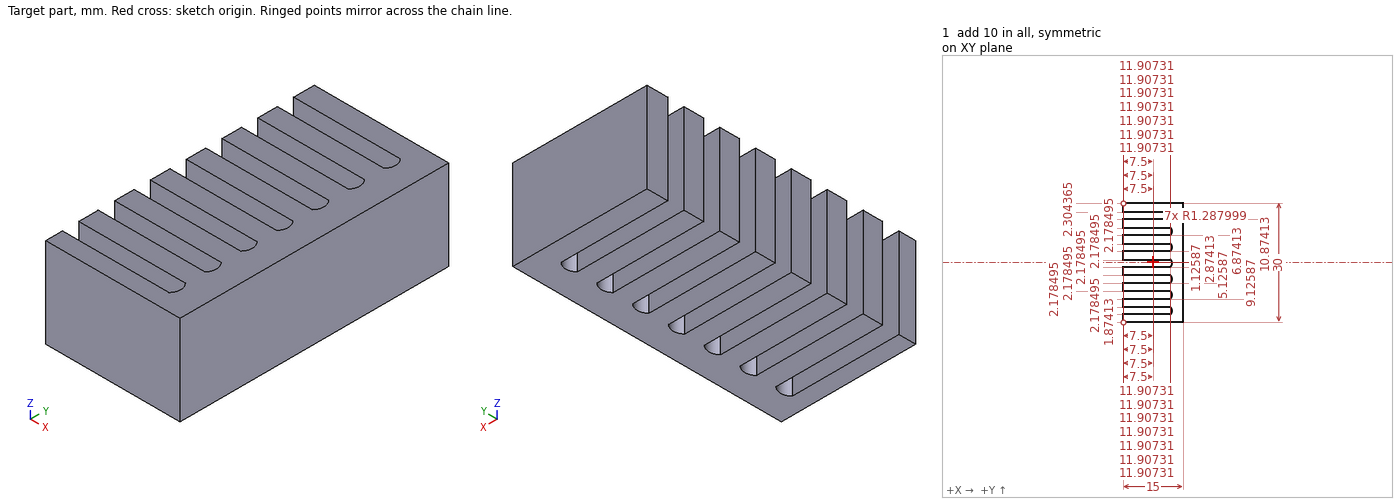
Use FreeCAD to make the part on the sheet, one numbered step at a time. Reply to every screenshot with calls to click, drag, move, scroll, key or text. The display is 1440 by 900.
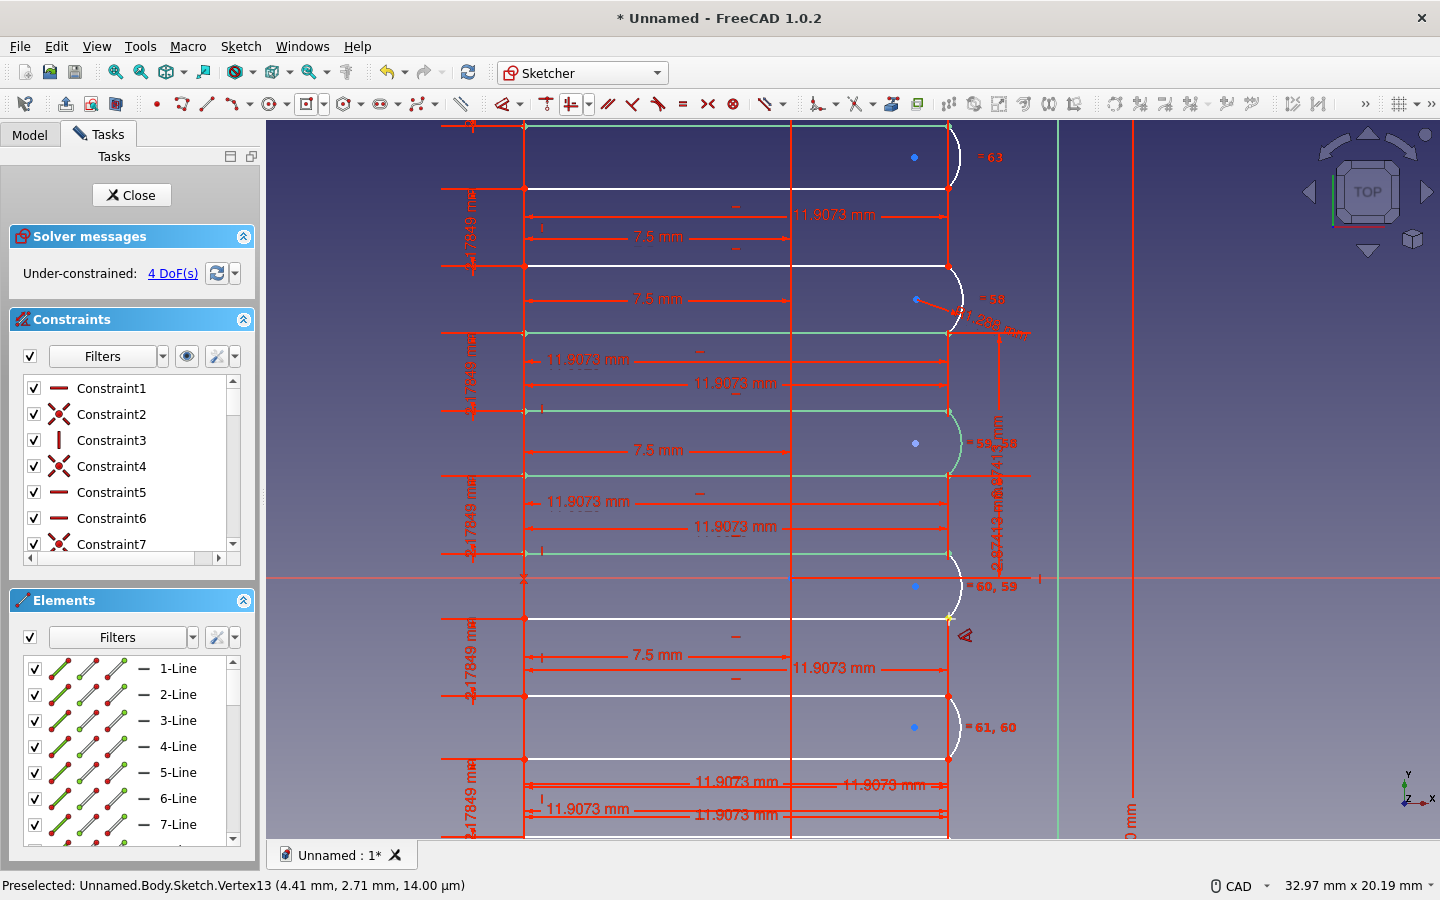
click(948, 619)
click(982, 598)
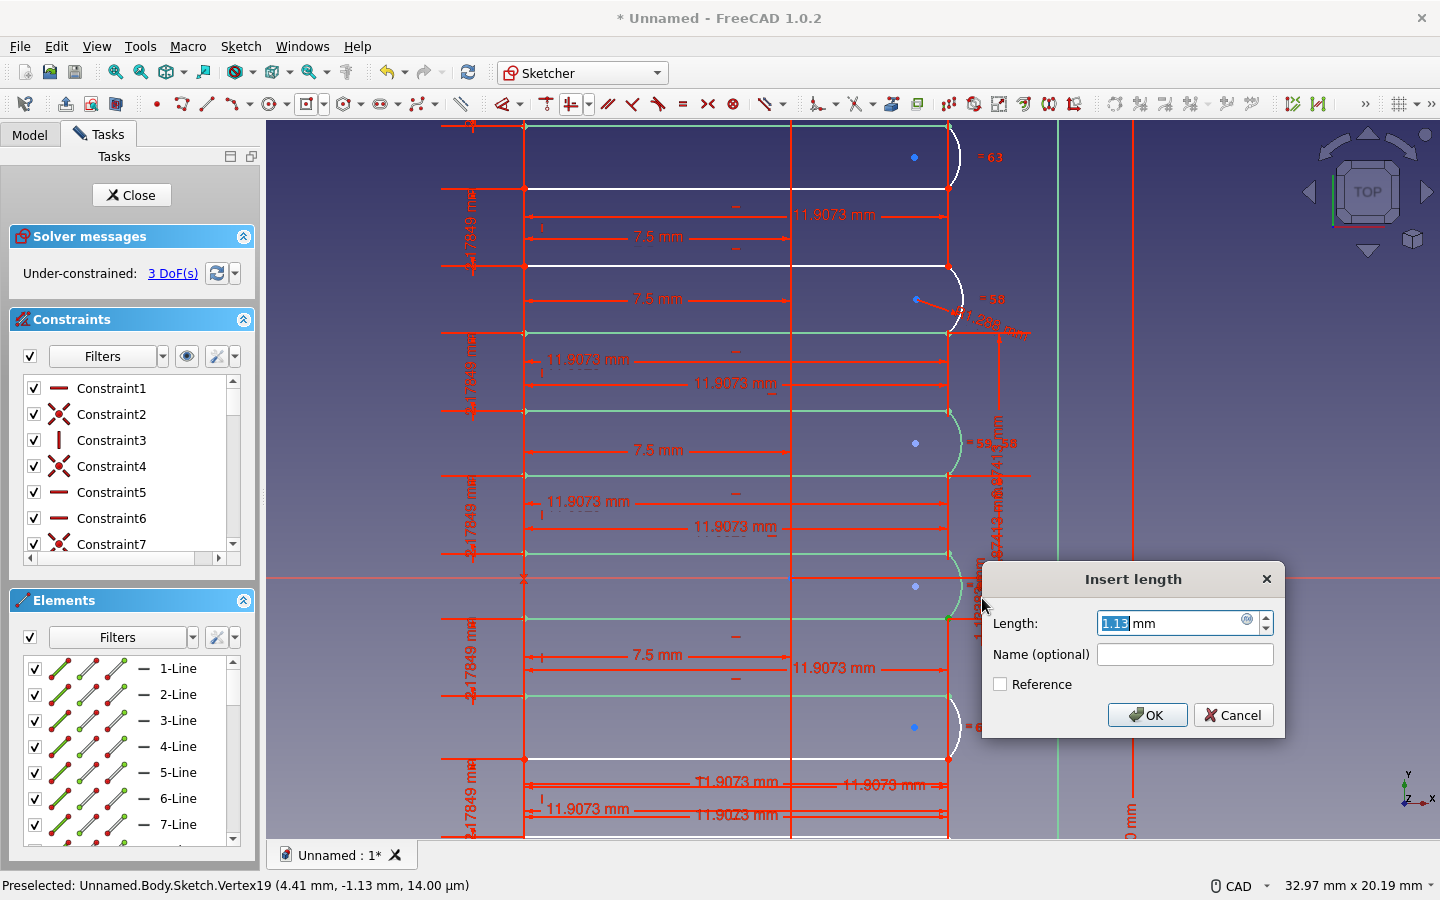
text(1.12587)
key(Return)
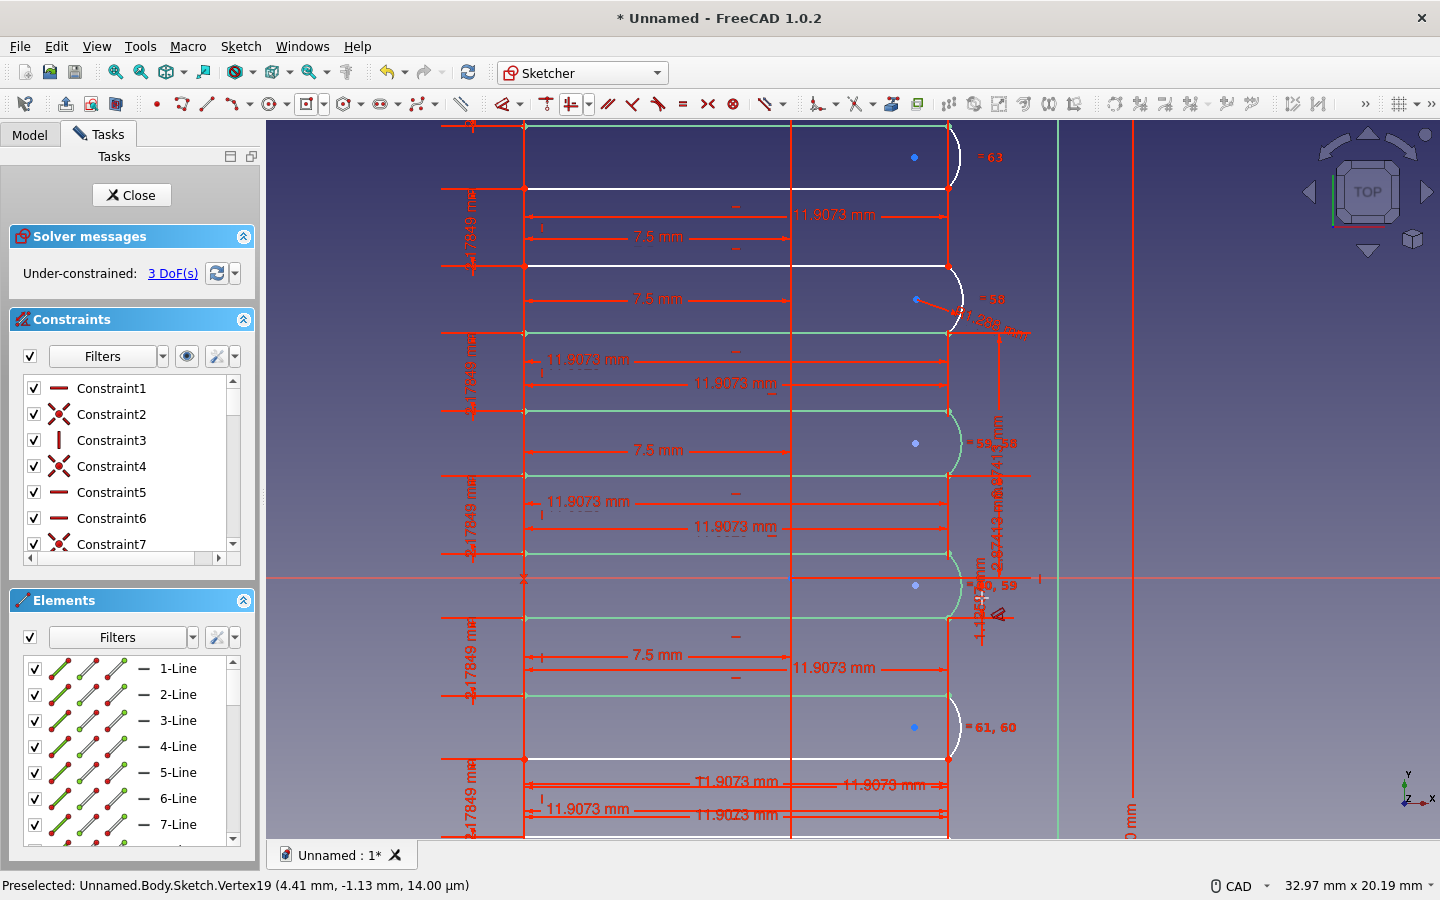
click(948, 759)
click(982, 669)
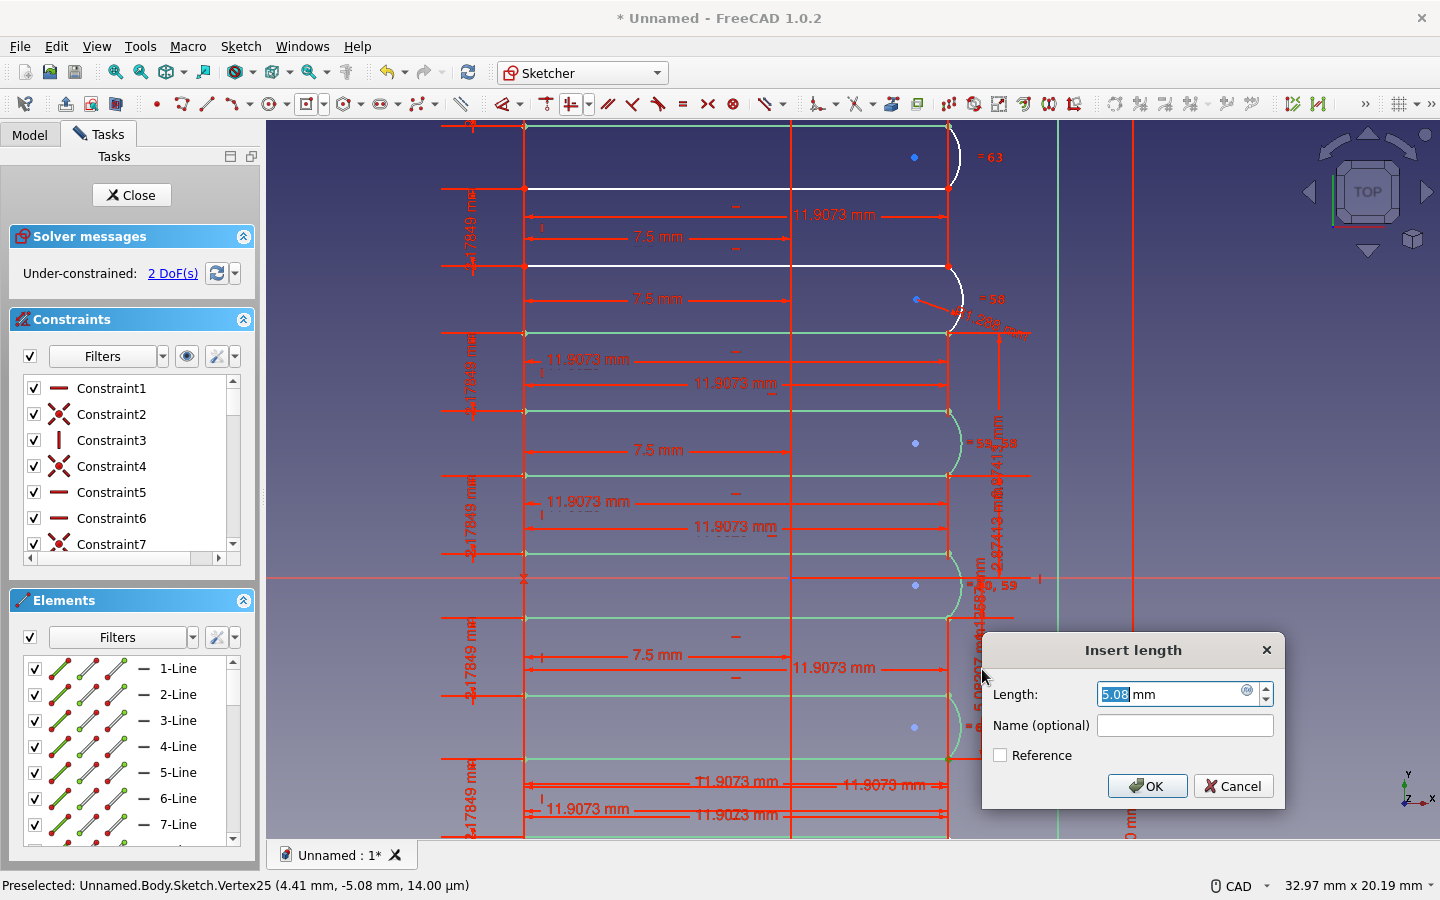
text(5.12587)
key(Return)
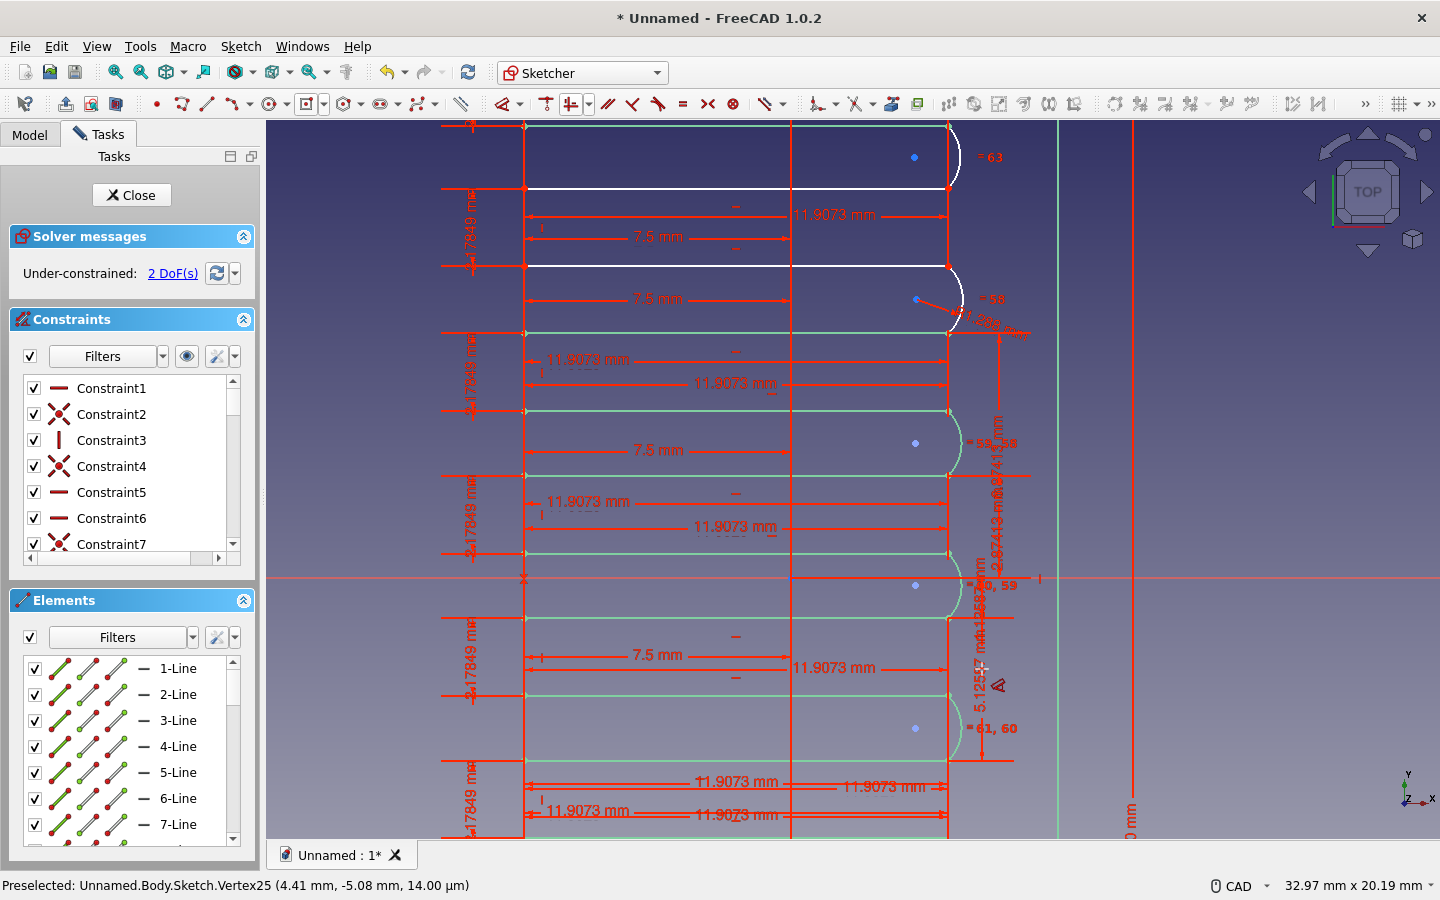
scroll(779, 399, down, 4)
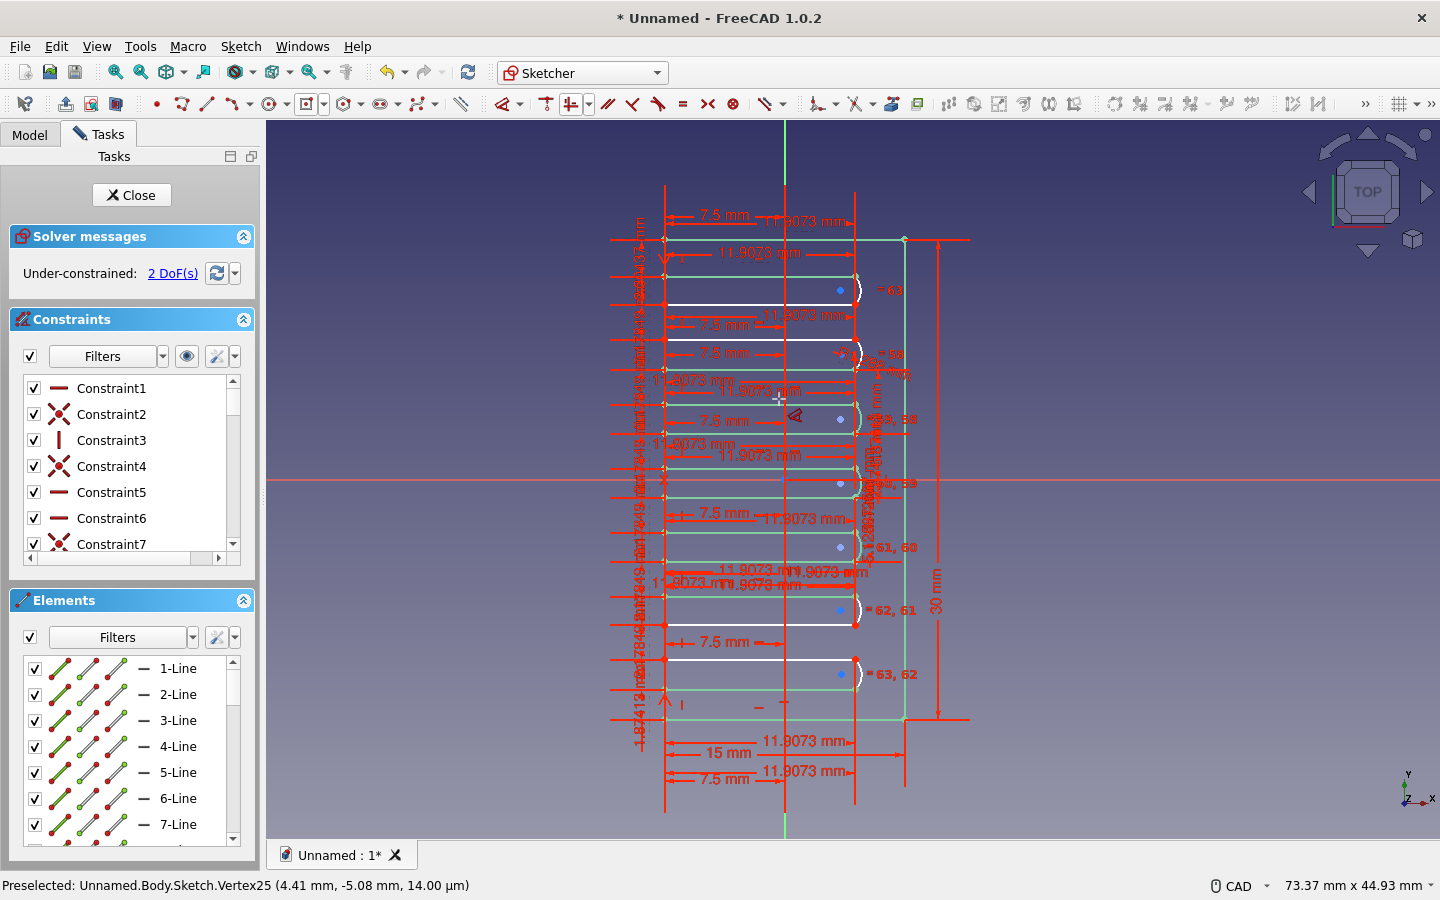
click(855, 625)
click(889, 552)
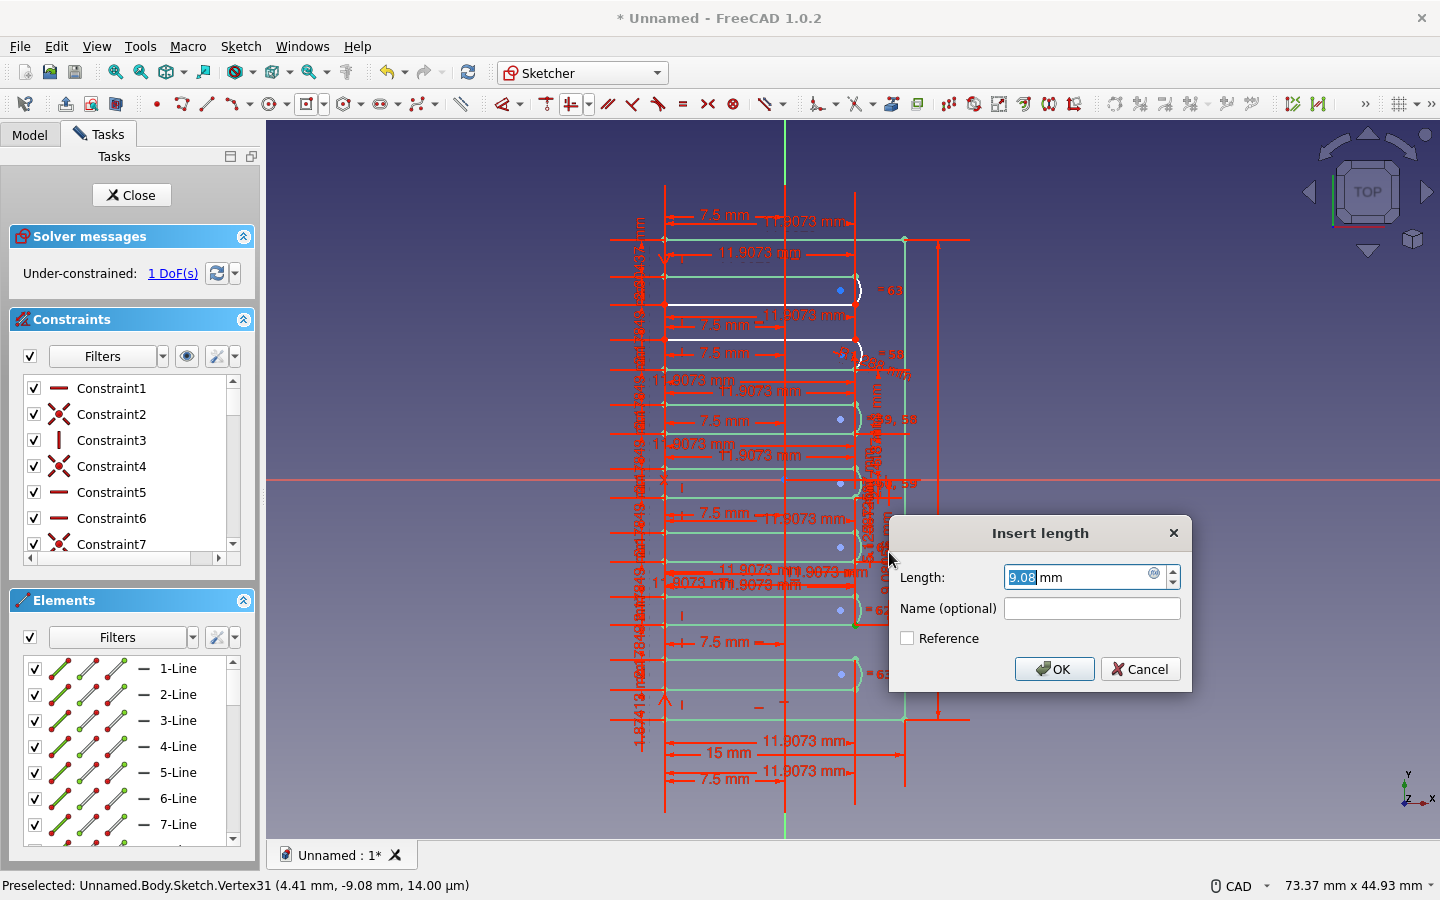
text(9.12587)
key(Return)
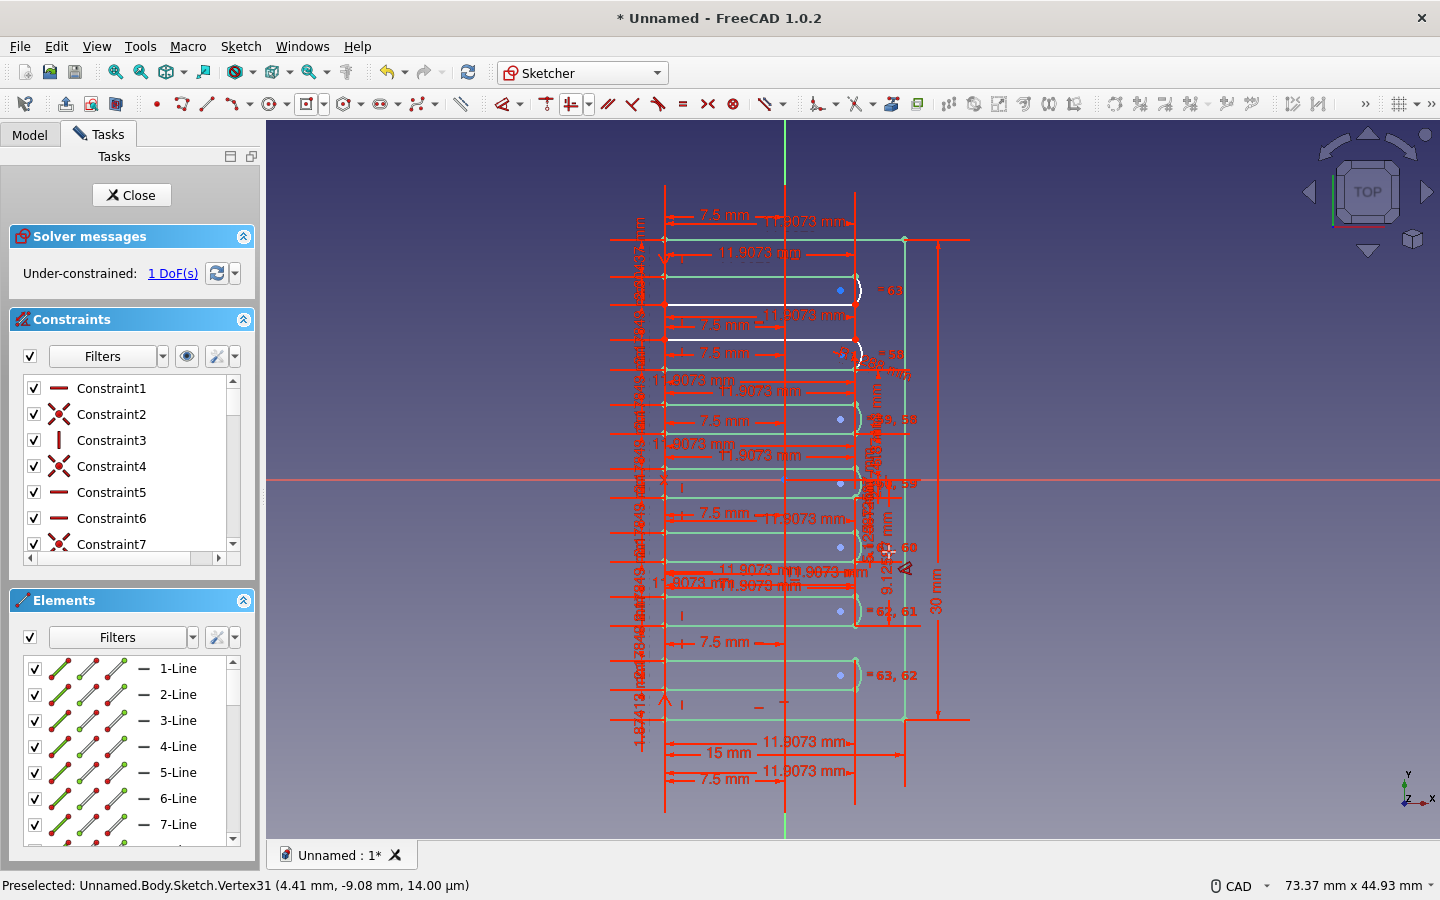
click(855, 305)
click(889, 392)